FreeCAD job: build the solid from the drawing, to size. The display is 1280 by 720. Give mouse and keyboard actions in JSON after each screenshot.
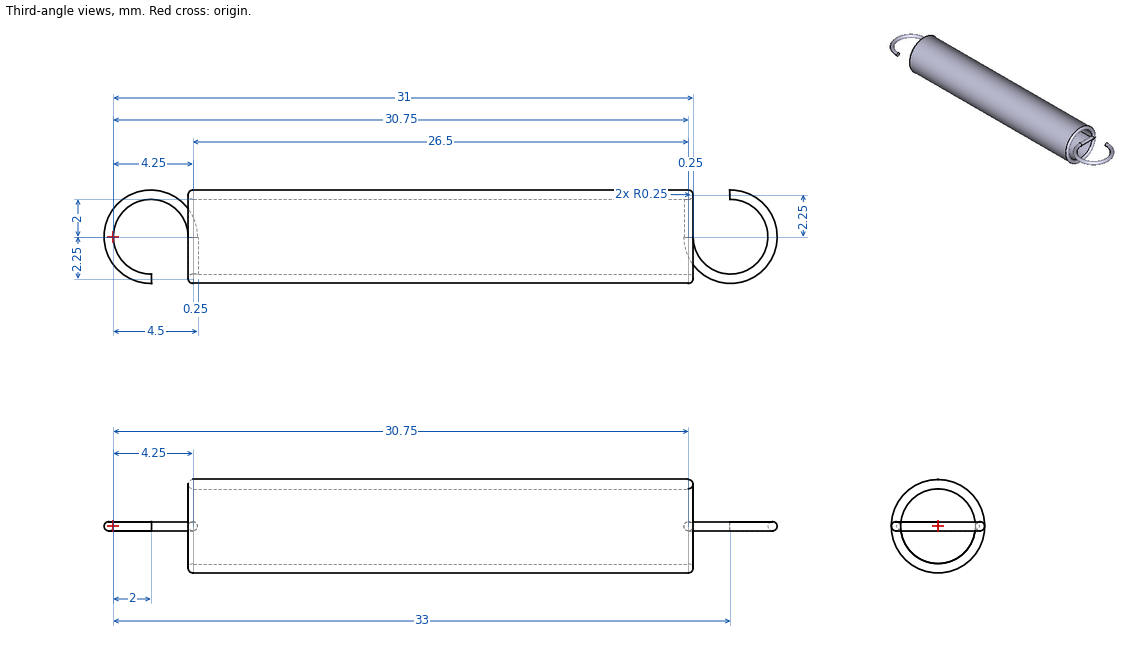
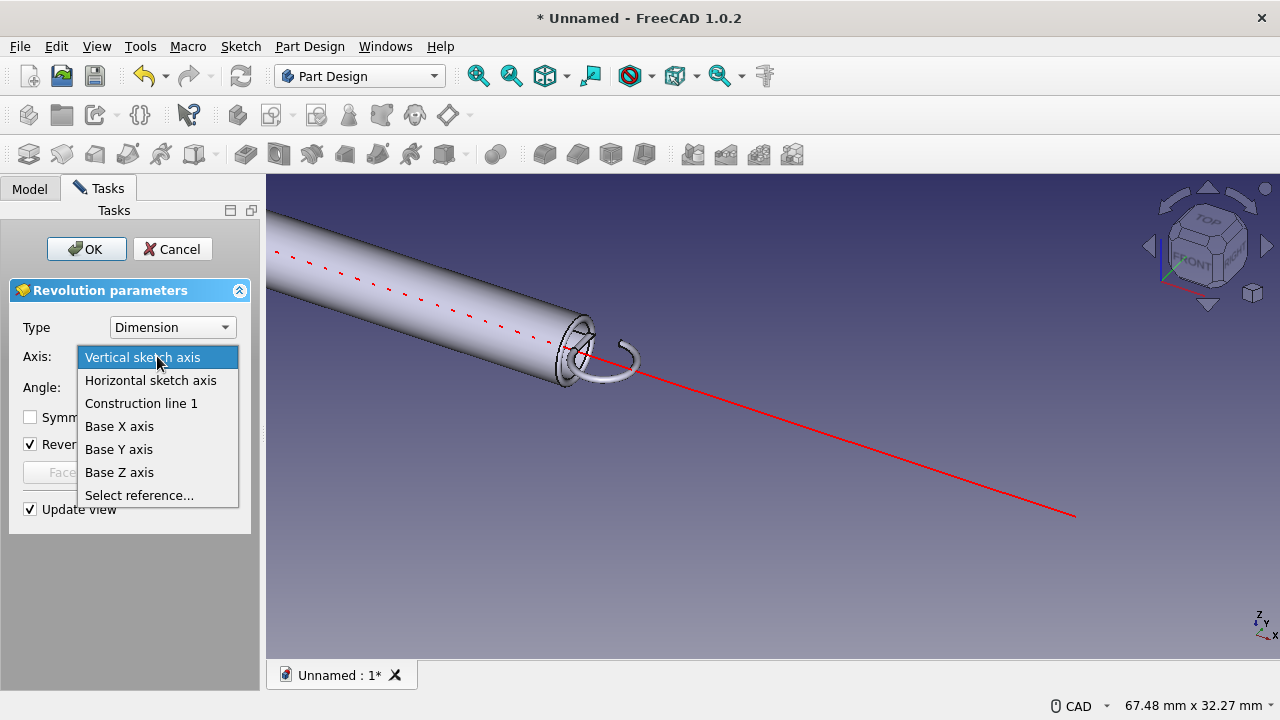
{"action": "left_click", "coordinate": [156, 404]}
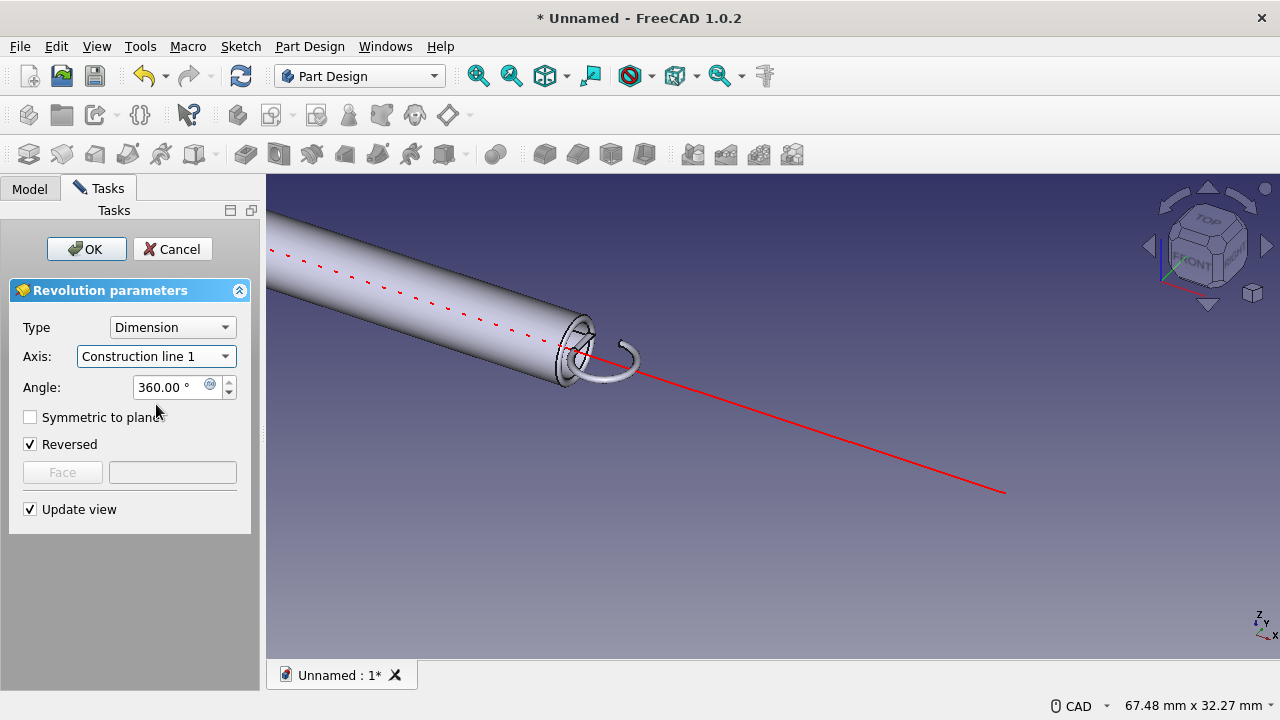
{"action": "left_click", "coordinate": [87, 249]}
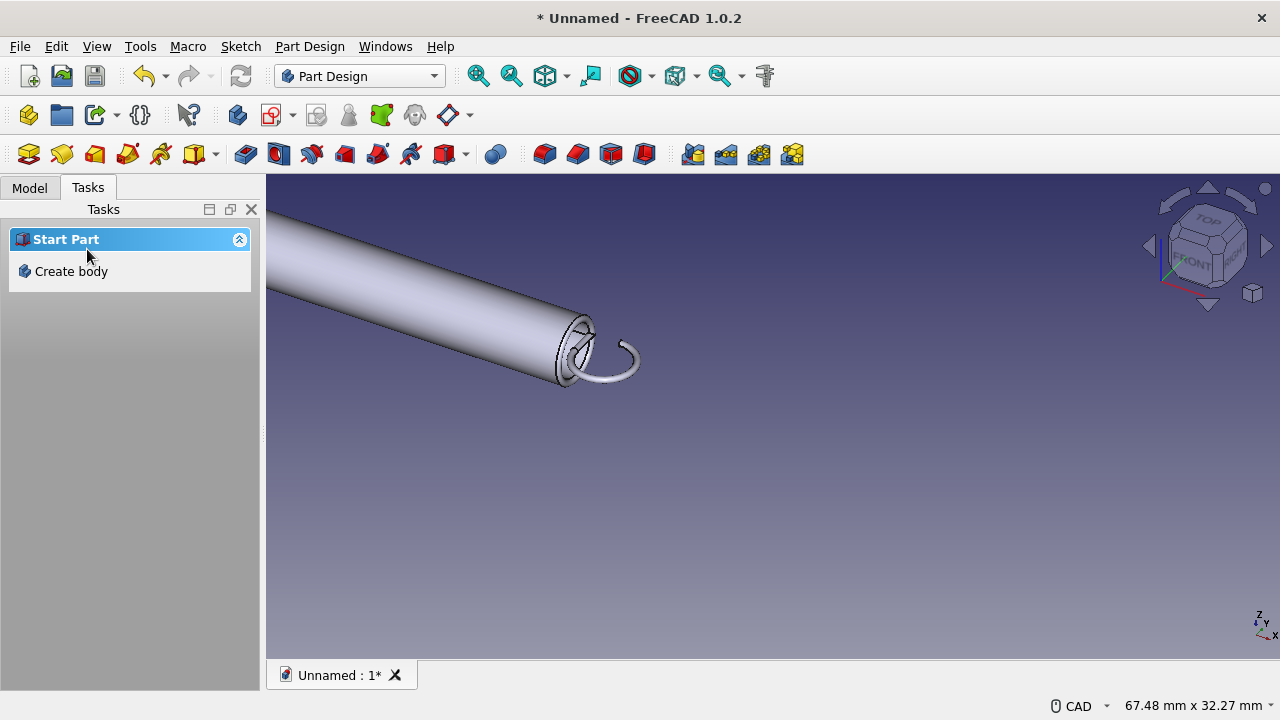
{"action": "key", "text": "v f"}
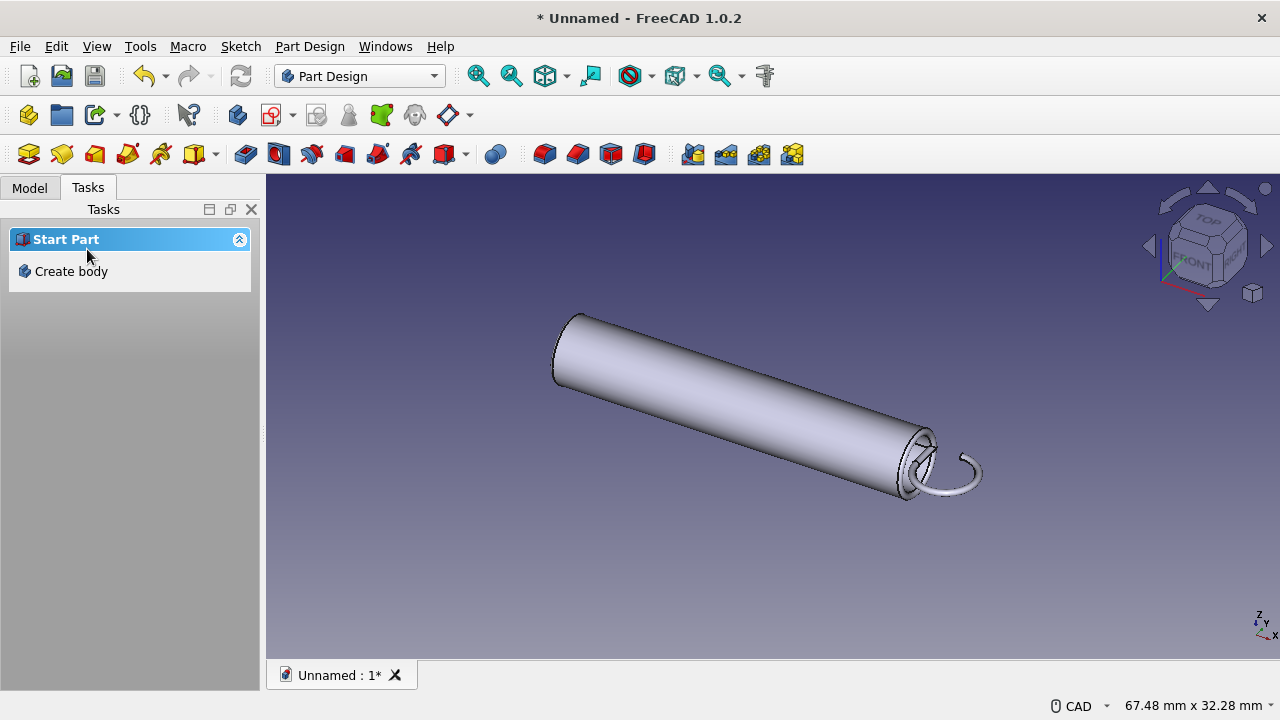
{"action": "left_click", "coordinate": [270, 116]}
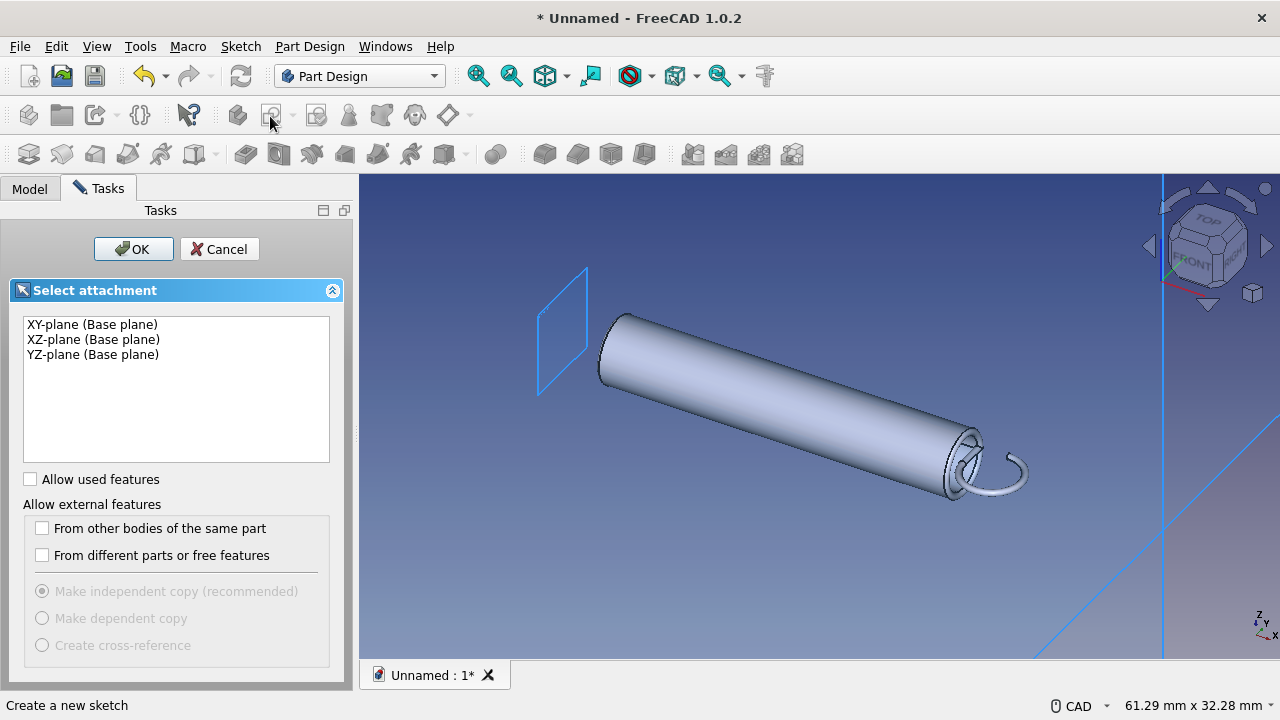
{"action": "left_click", "coordinate": [84, 340]}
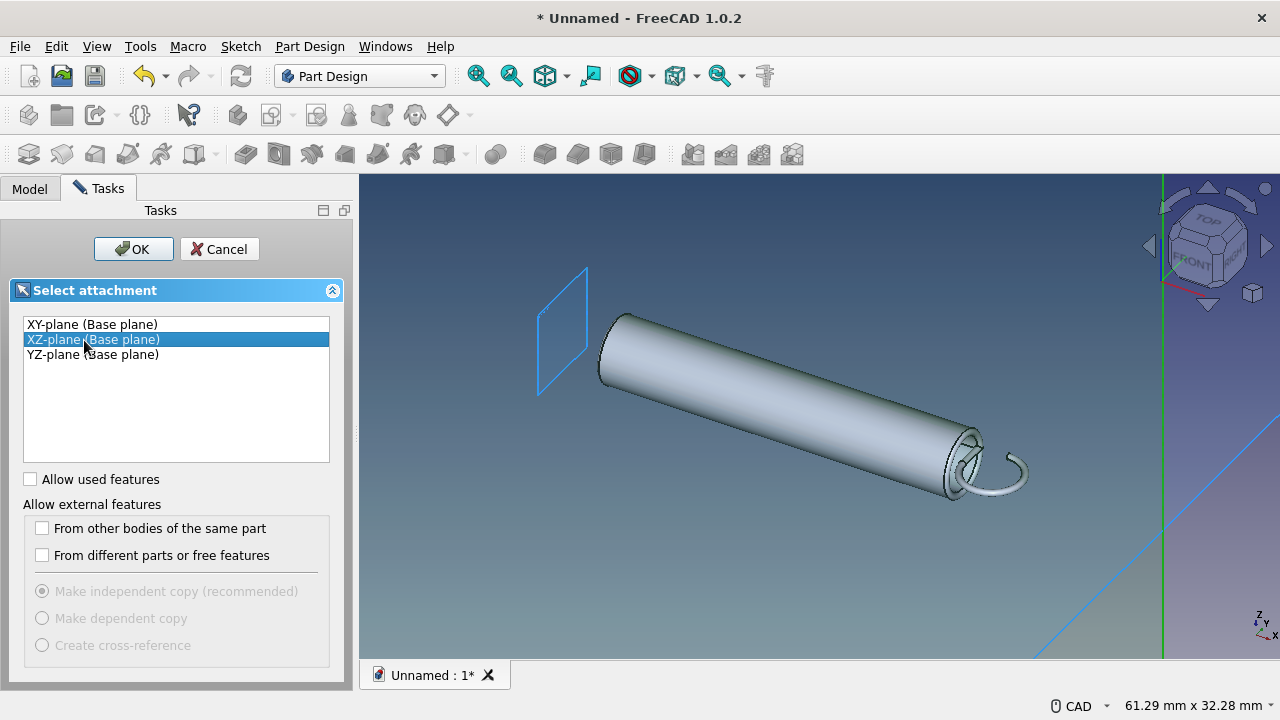
{"action": "left_click", "coordinate": [134, 249]}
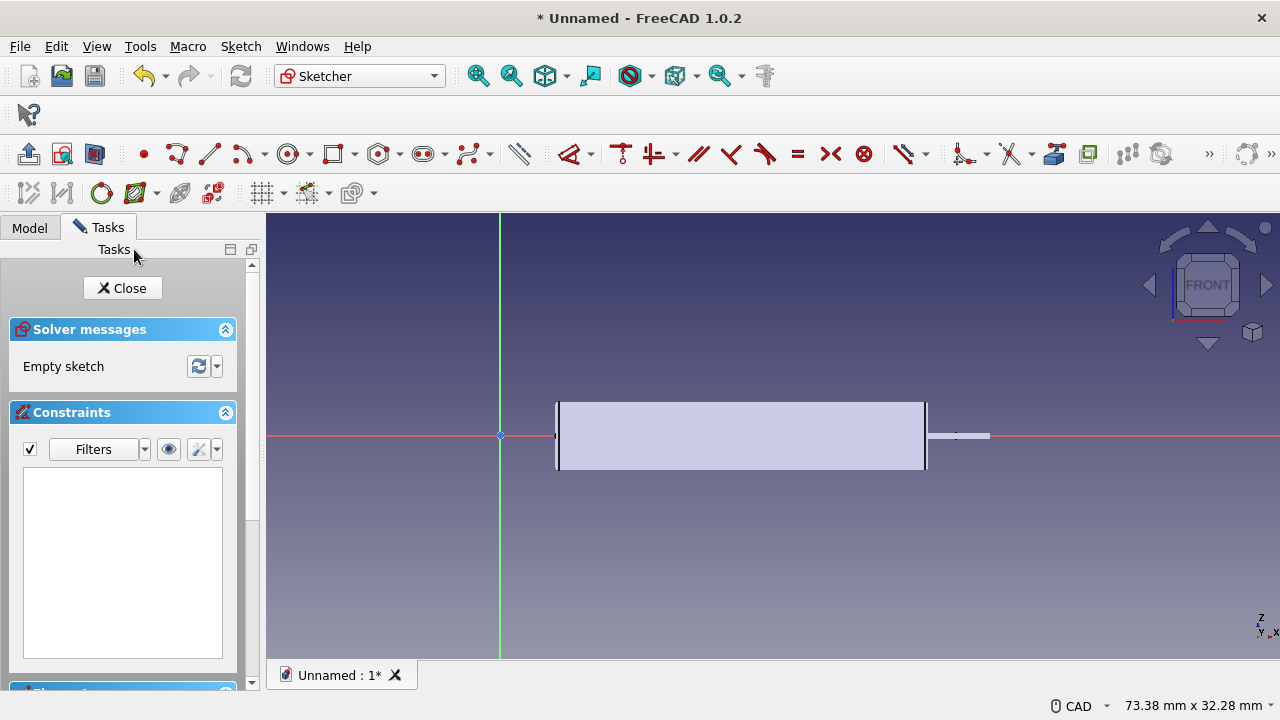
{"action": "key", "text": "q s"}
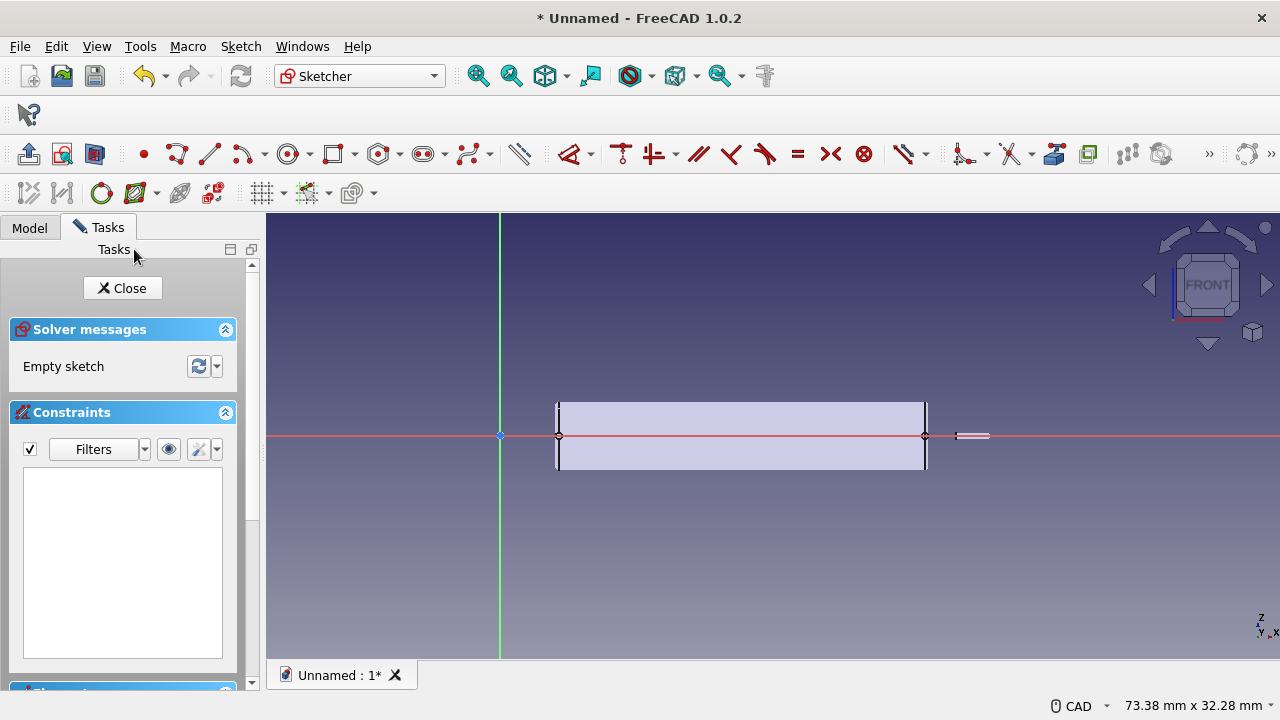
{"action": "scroll", "coordinate": [510, 436], "scroll_direction": "up", "scroll_amount": 11}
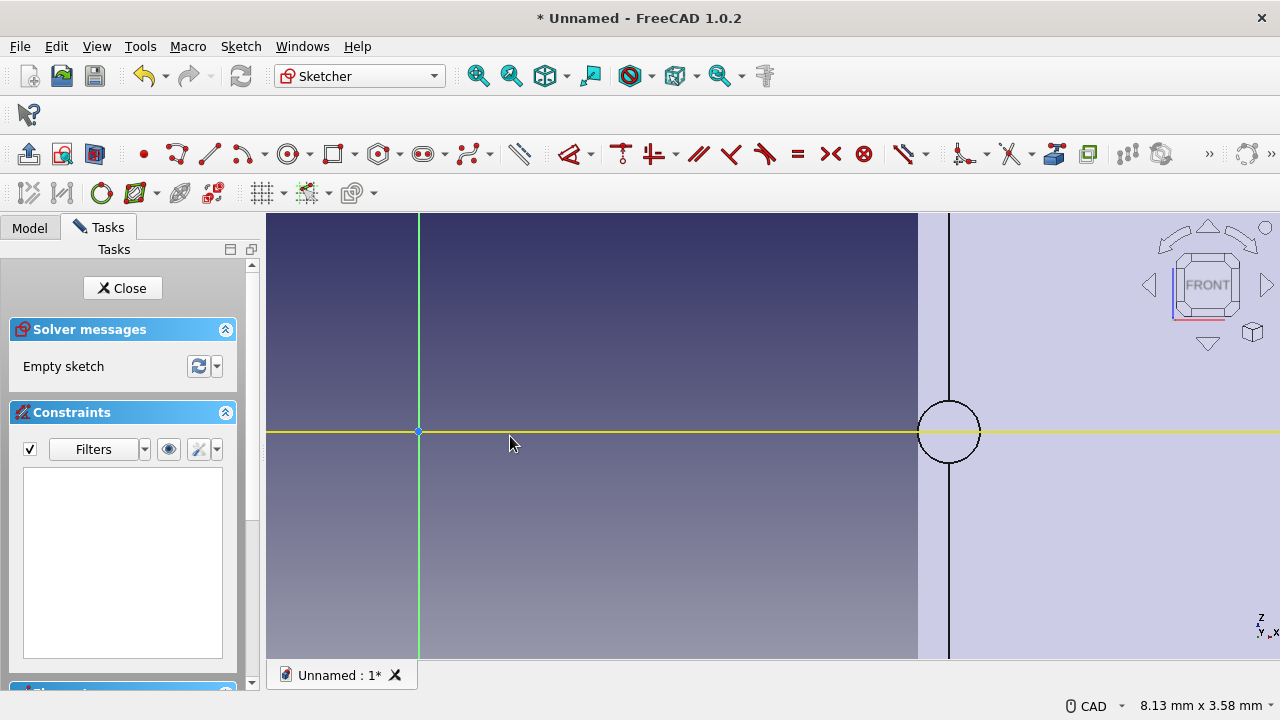
{"action": "key", "text": "g c"}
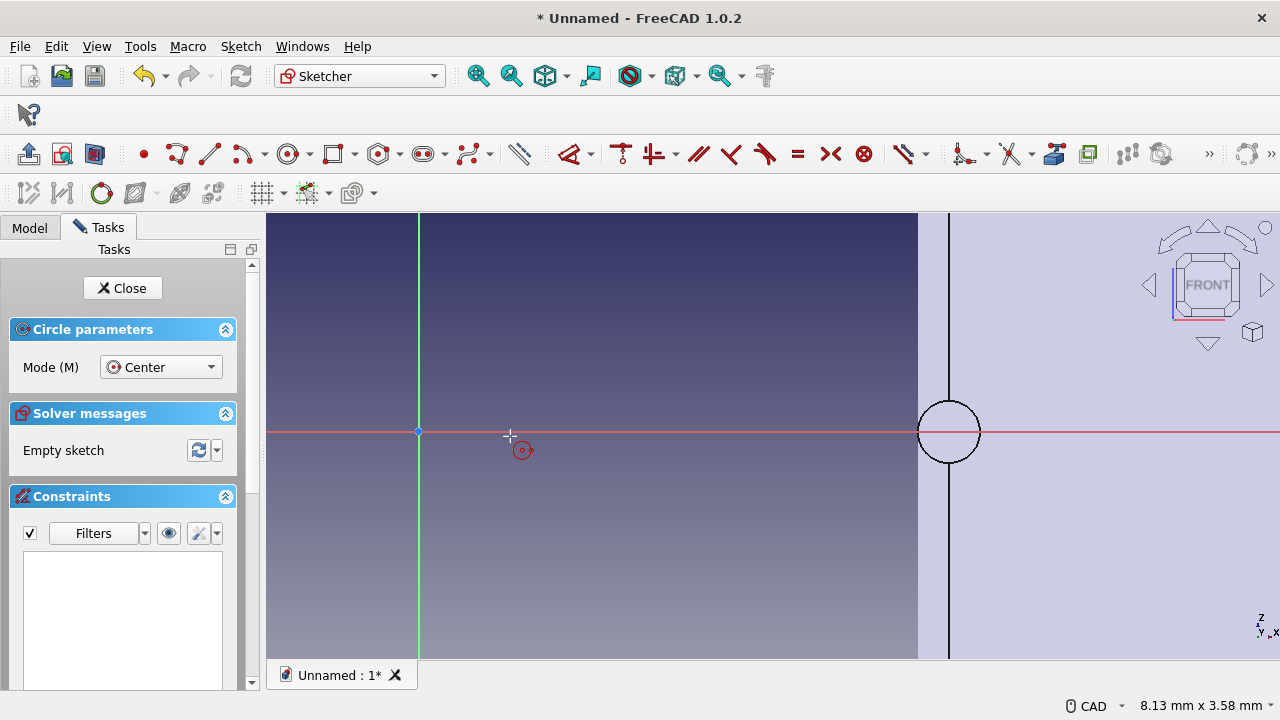
{"action": "left_click", "coordinate": [949, 432]}
{"action": "left_click", "coordinate": [971, 410]}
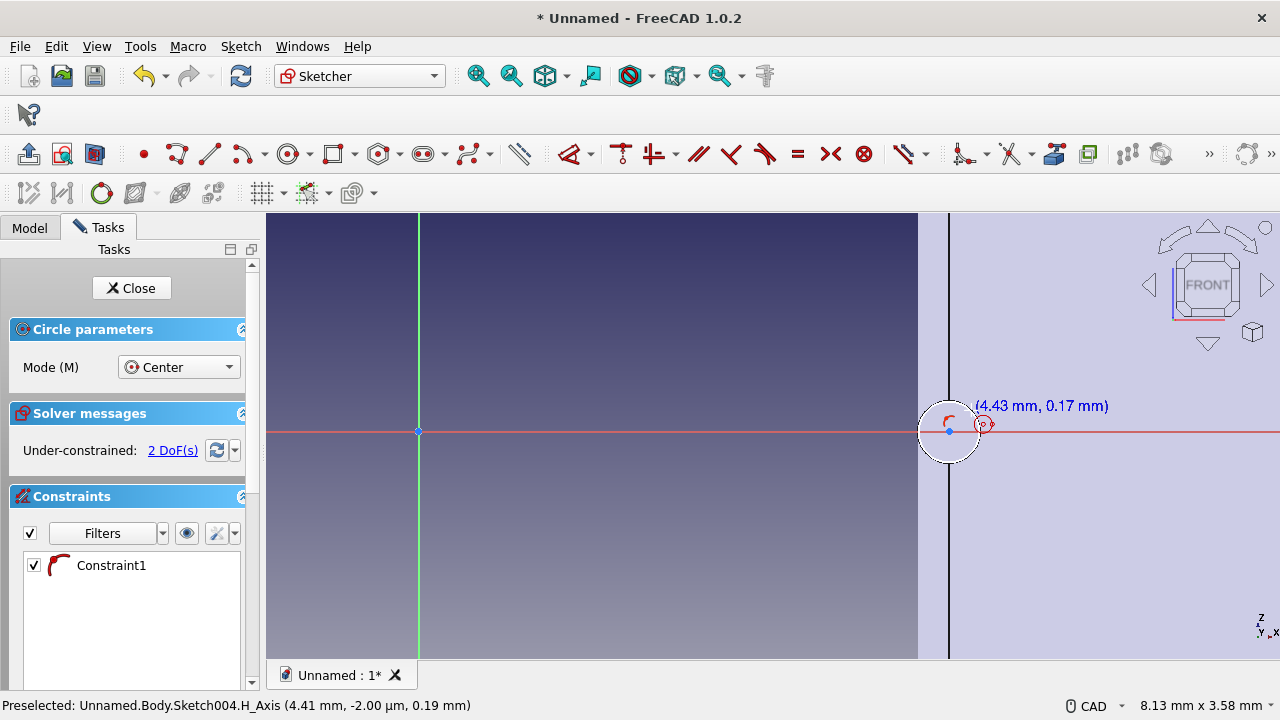
{"action": "left_click", "coordinate": [210, 154]}